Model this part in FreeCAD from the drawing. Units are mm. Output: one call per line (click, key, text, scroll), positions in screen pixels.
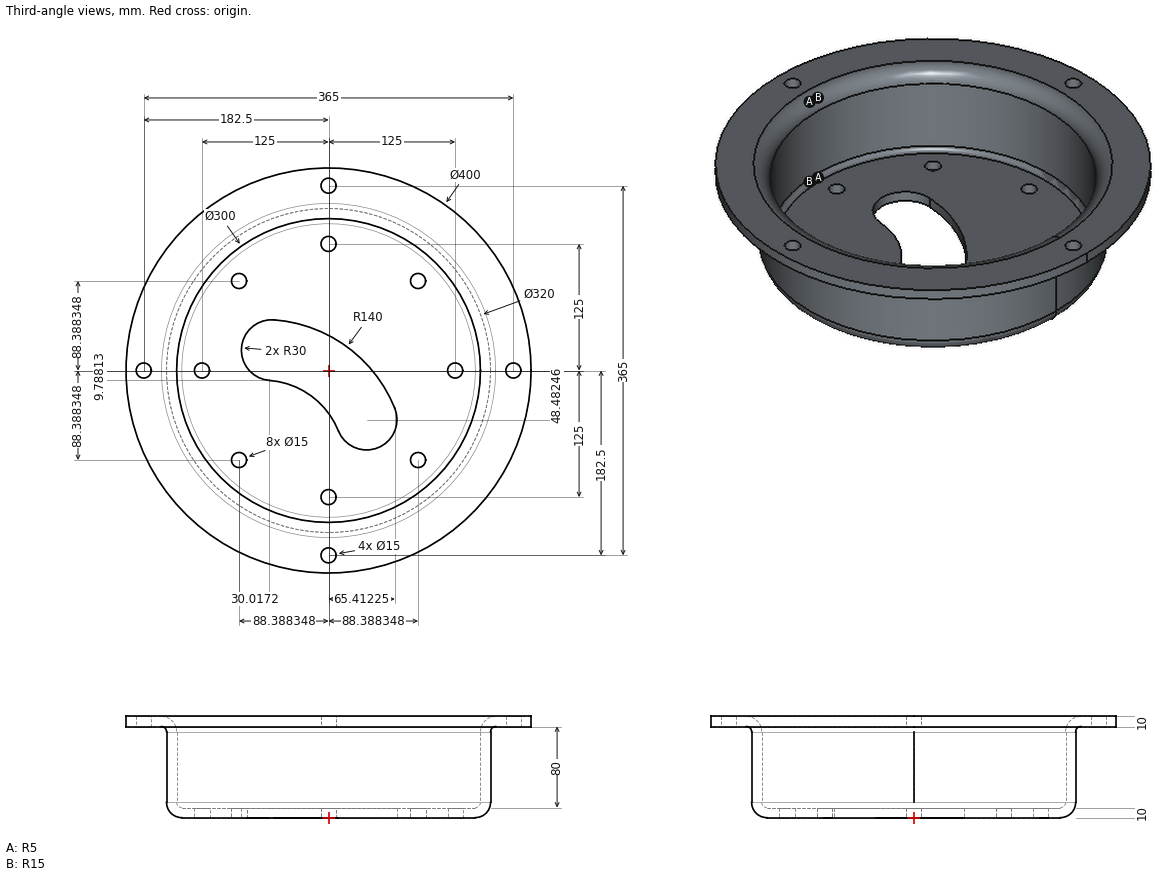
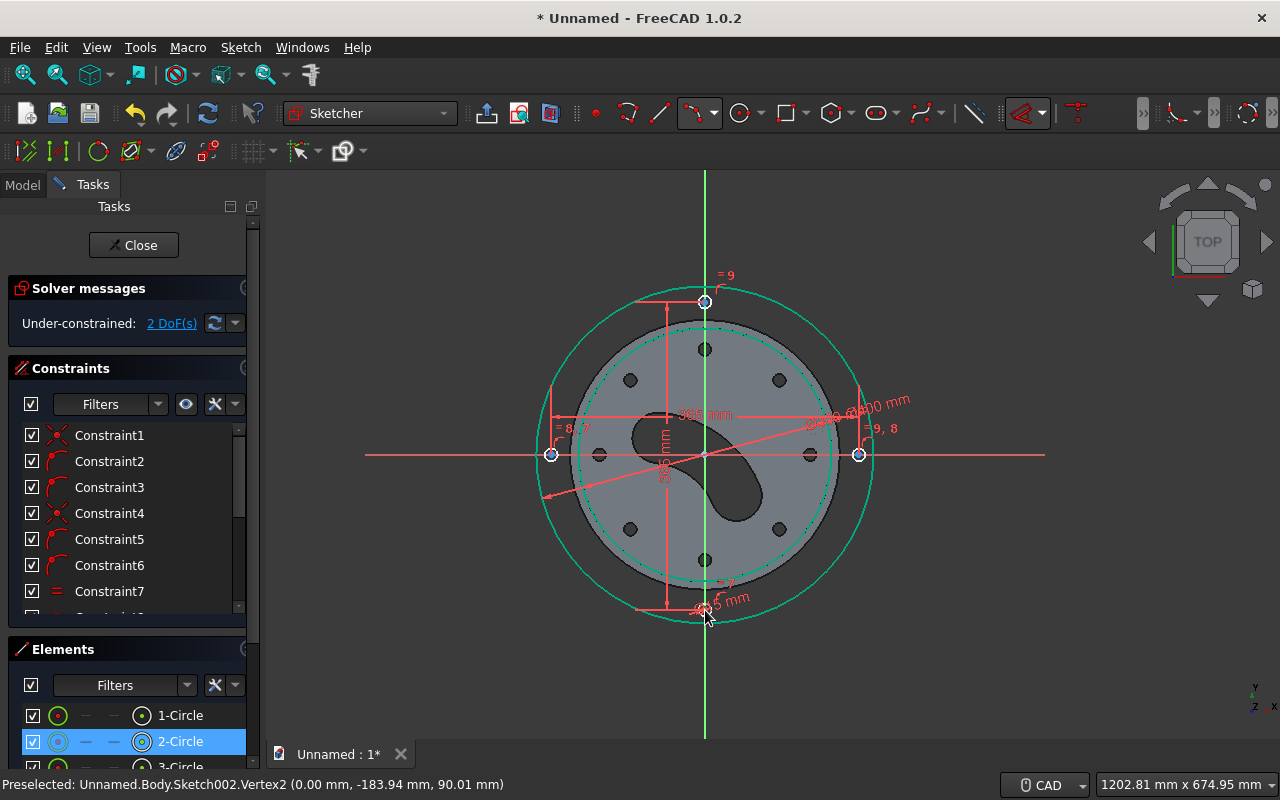
click(1044, 114)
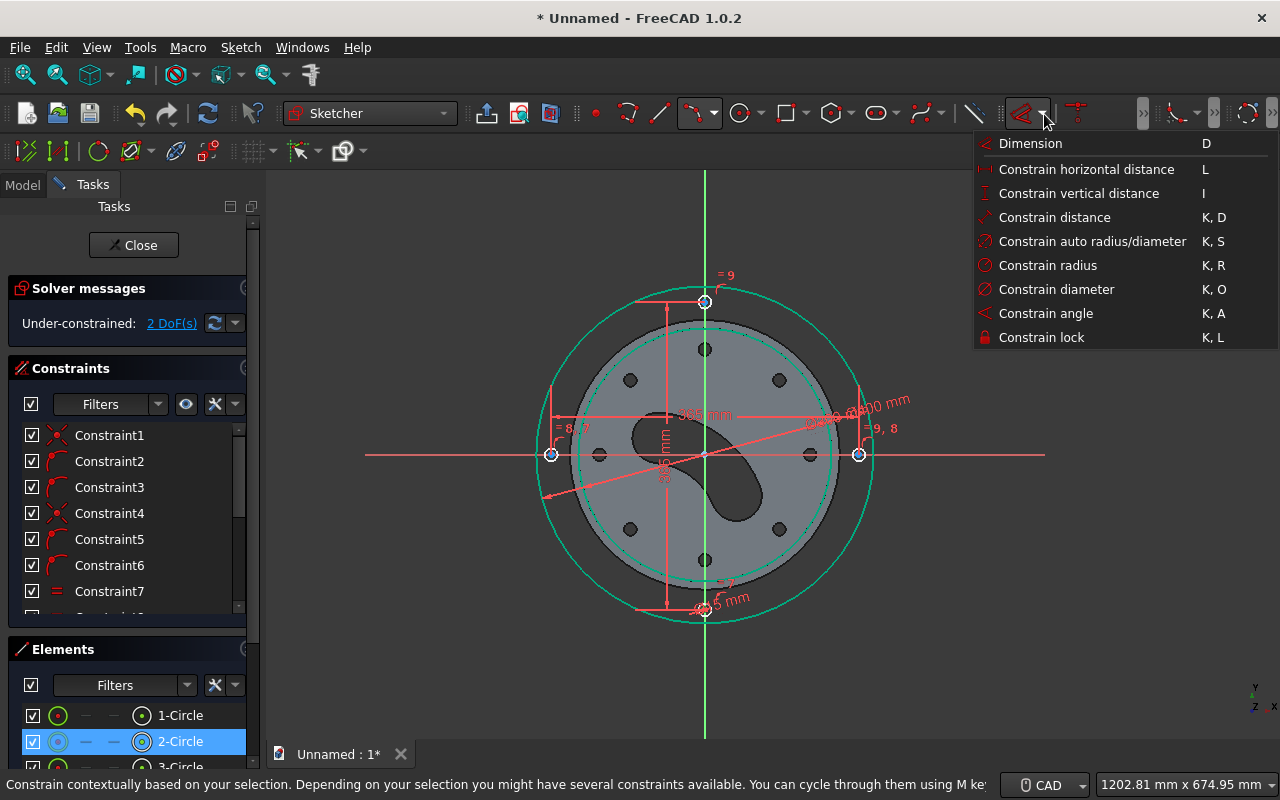
click(1126, 193)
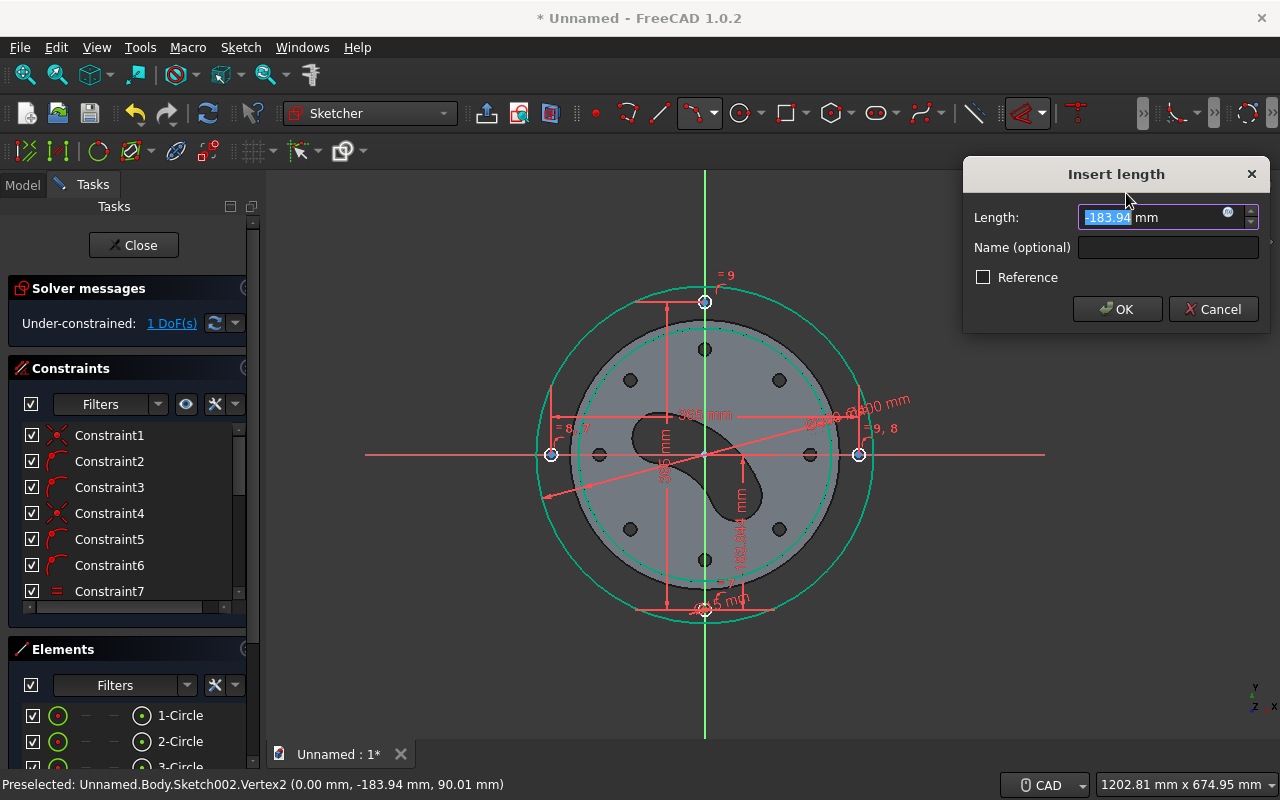
text(-182.5)
key(Return)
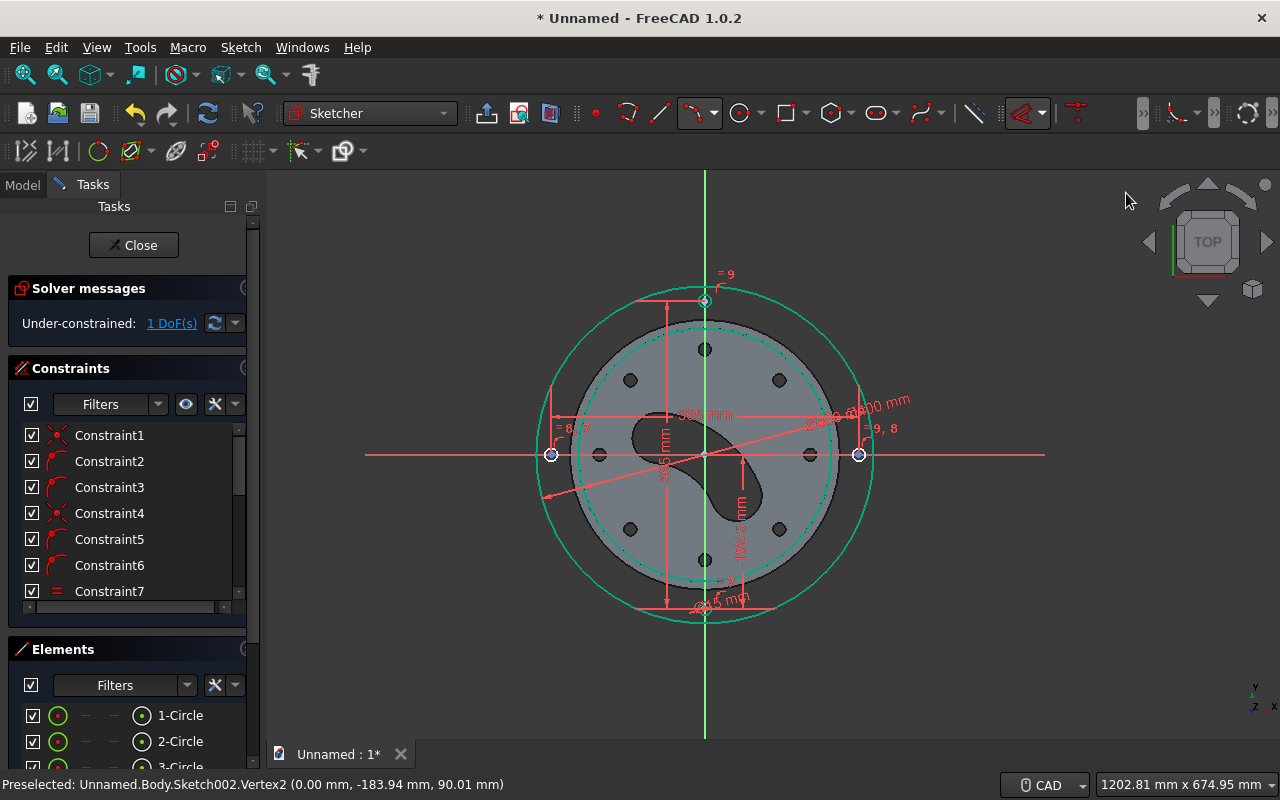
click(551, 455)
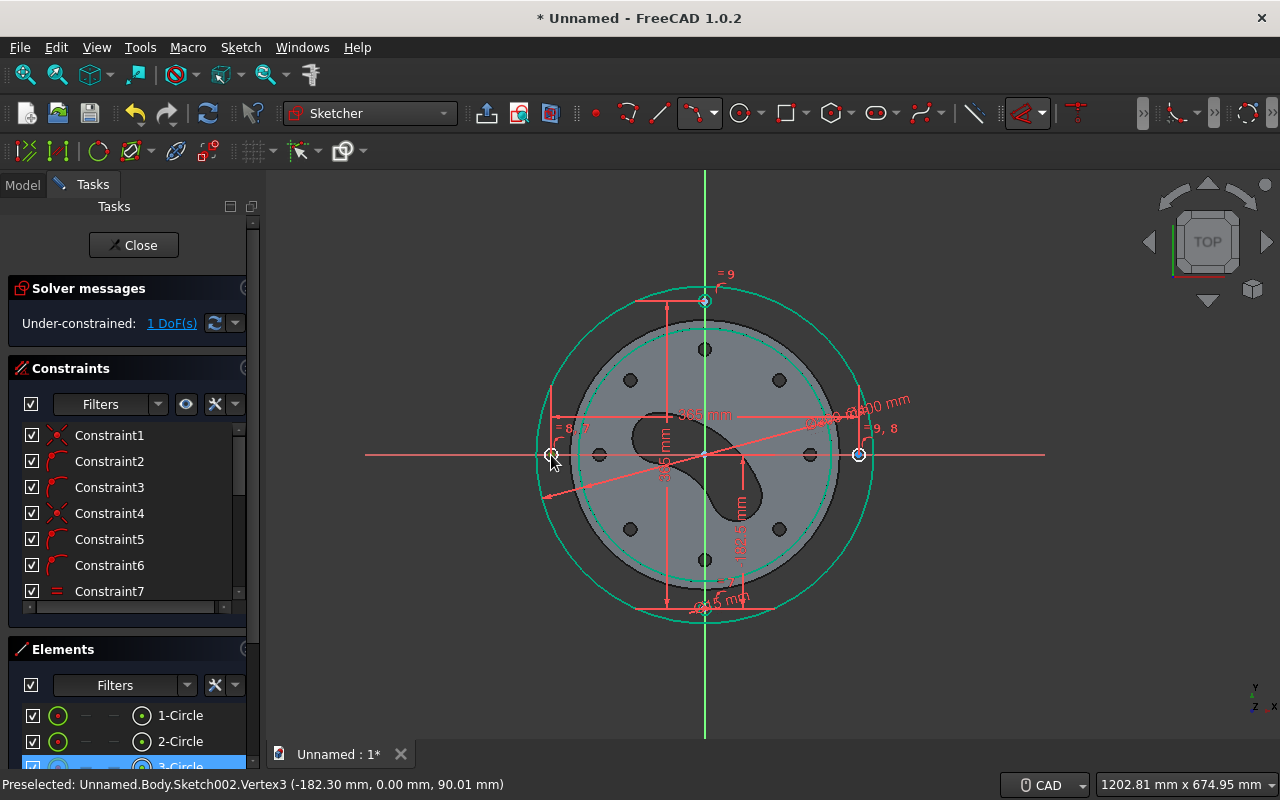
click(1044, 114)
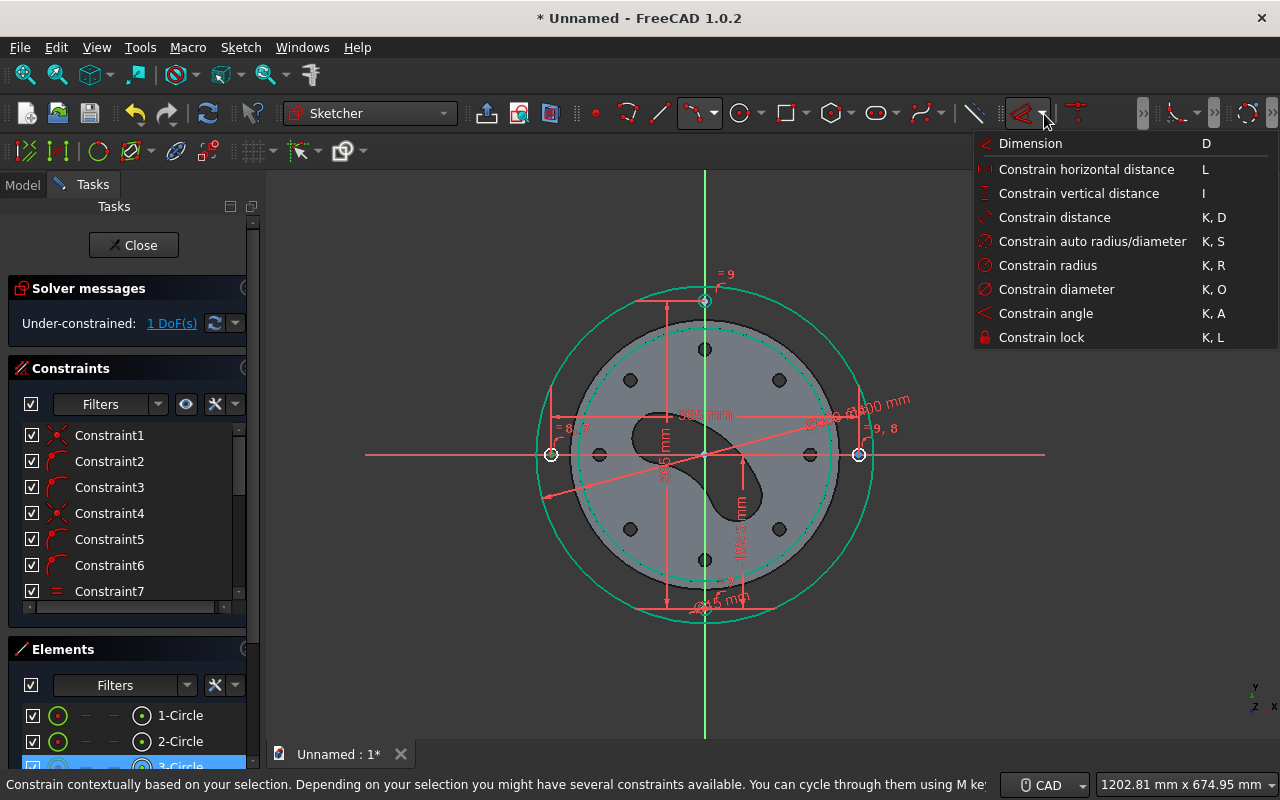
click(1126, 169)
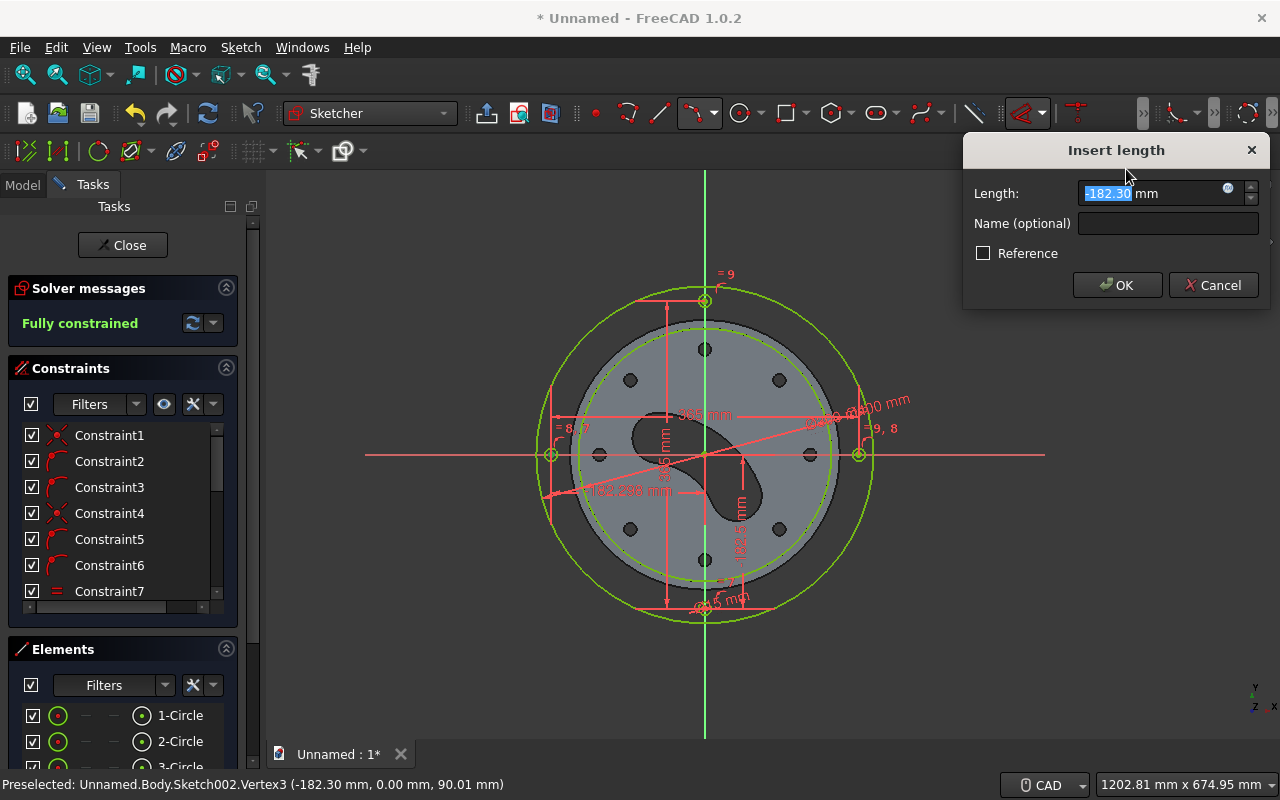
text(-182.5)
key(Return)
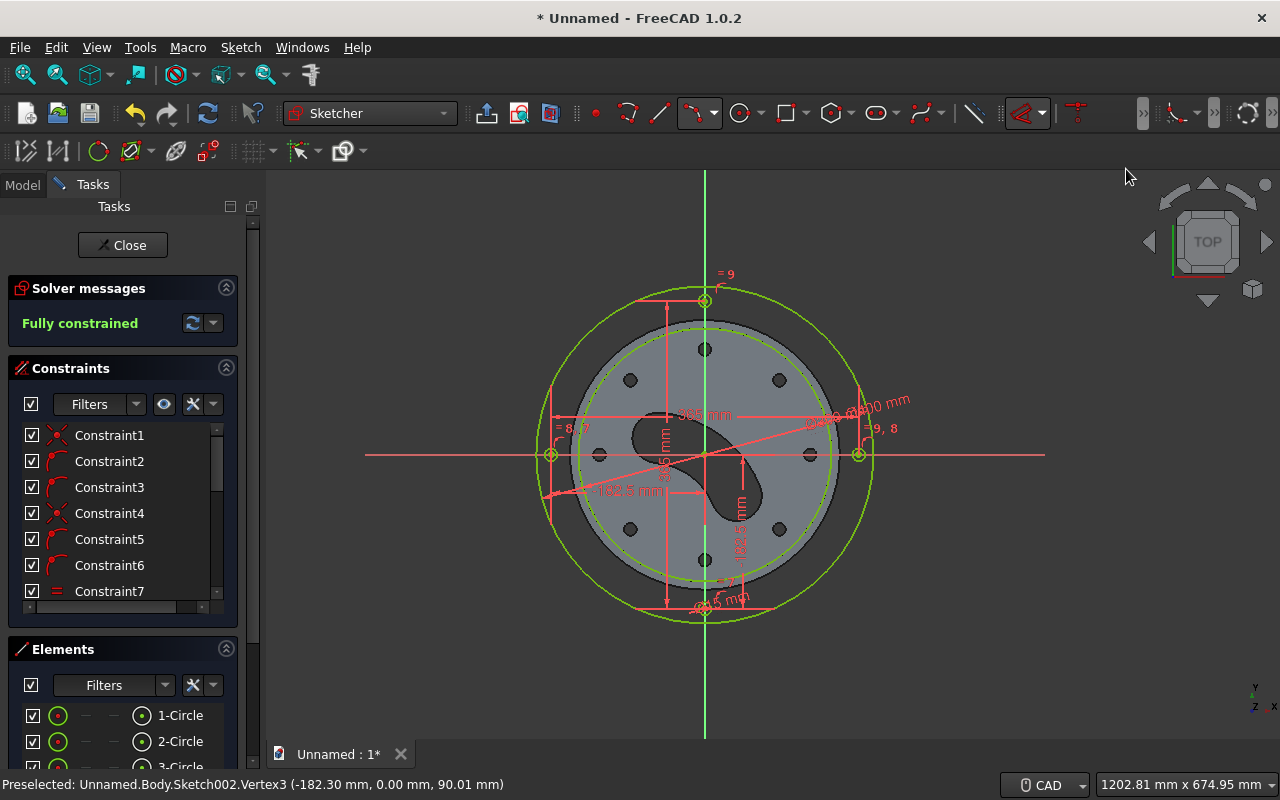
click(123, 245)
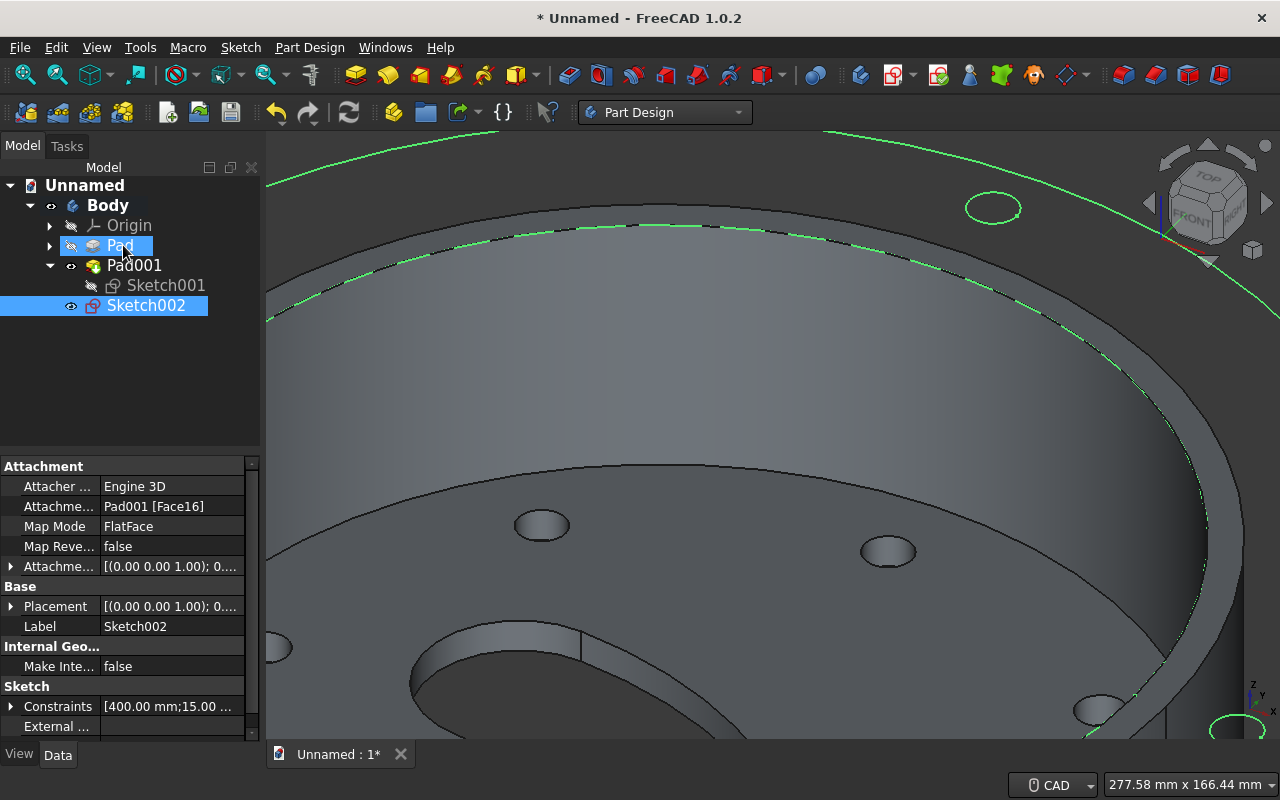
click(356, 76)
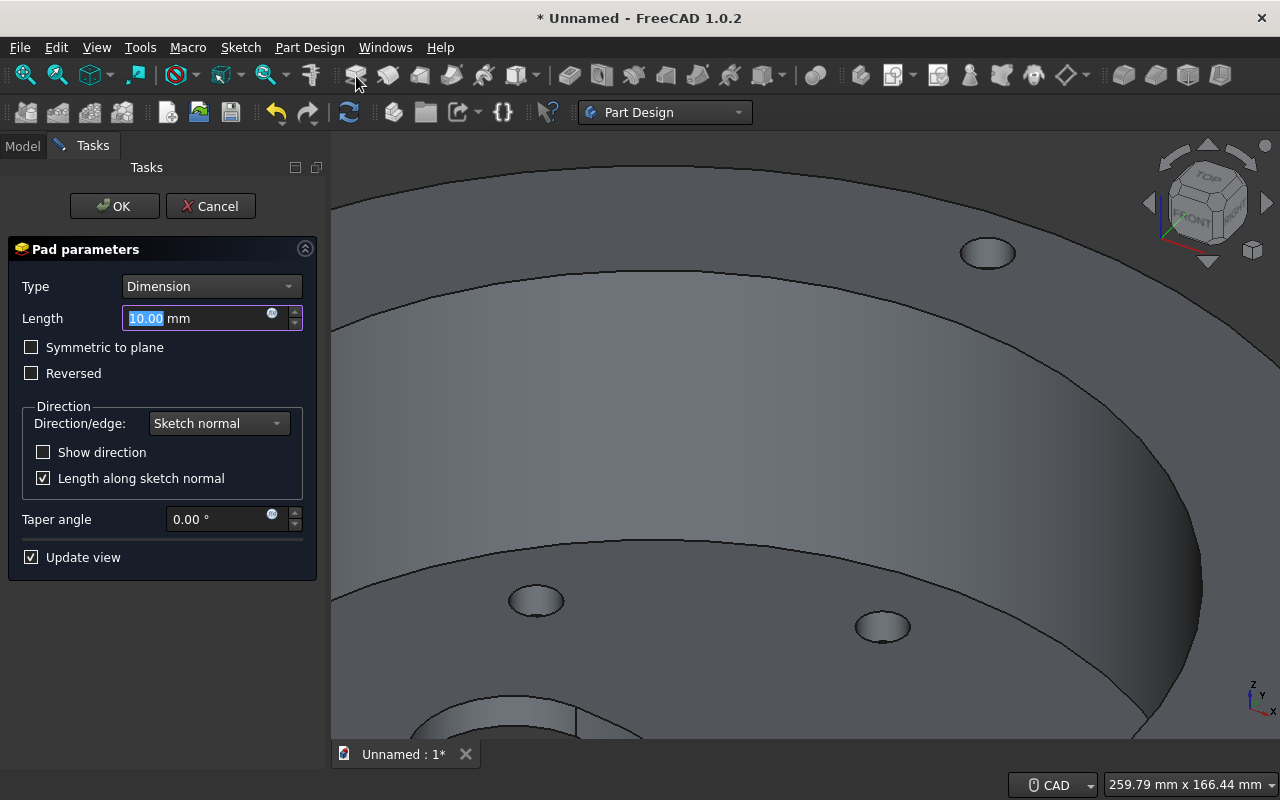
text(10)
key(Tab)